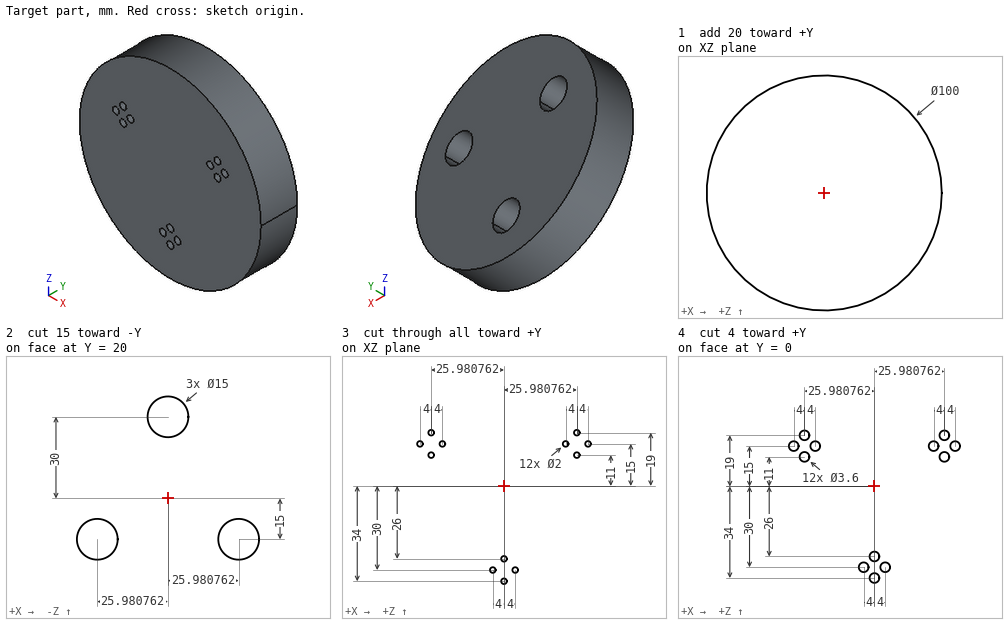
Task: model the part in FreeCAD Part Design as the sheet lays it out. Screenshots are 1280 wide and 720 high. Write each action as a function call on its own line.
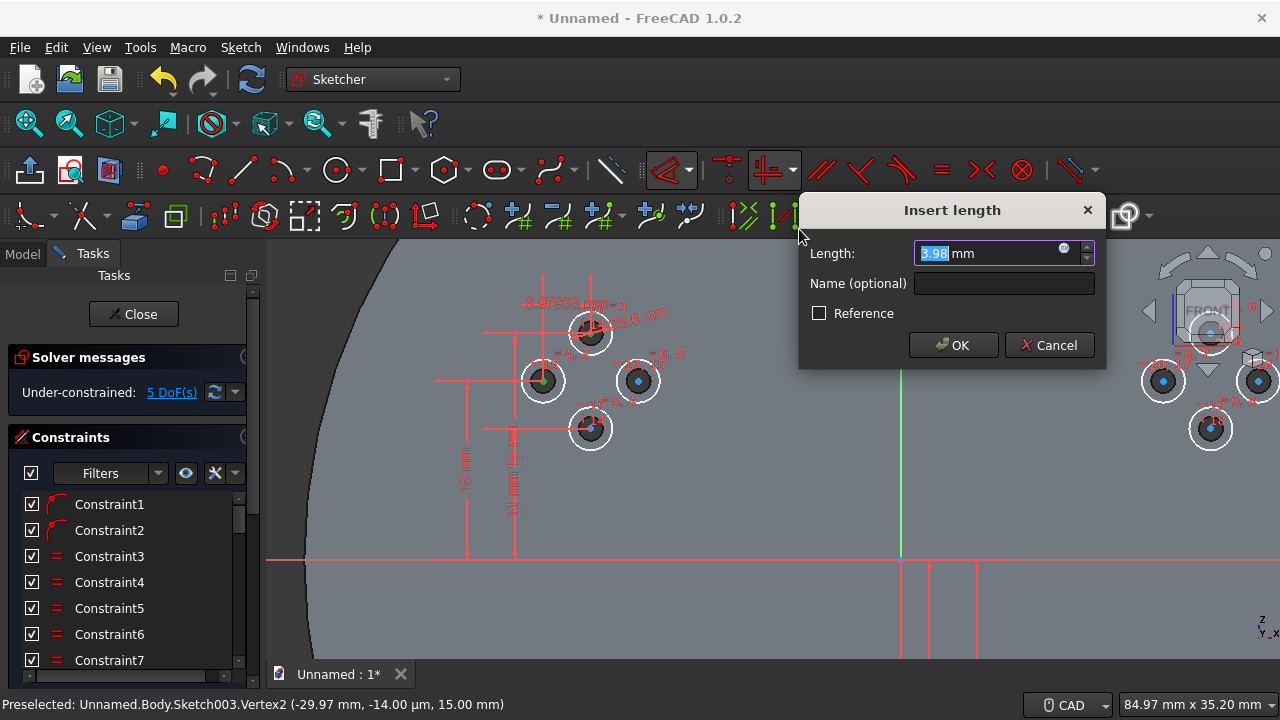
text(4)
key(Return)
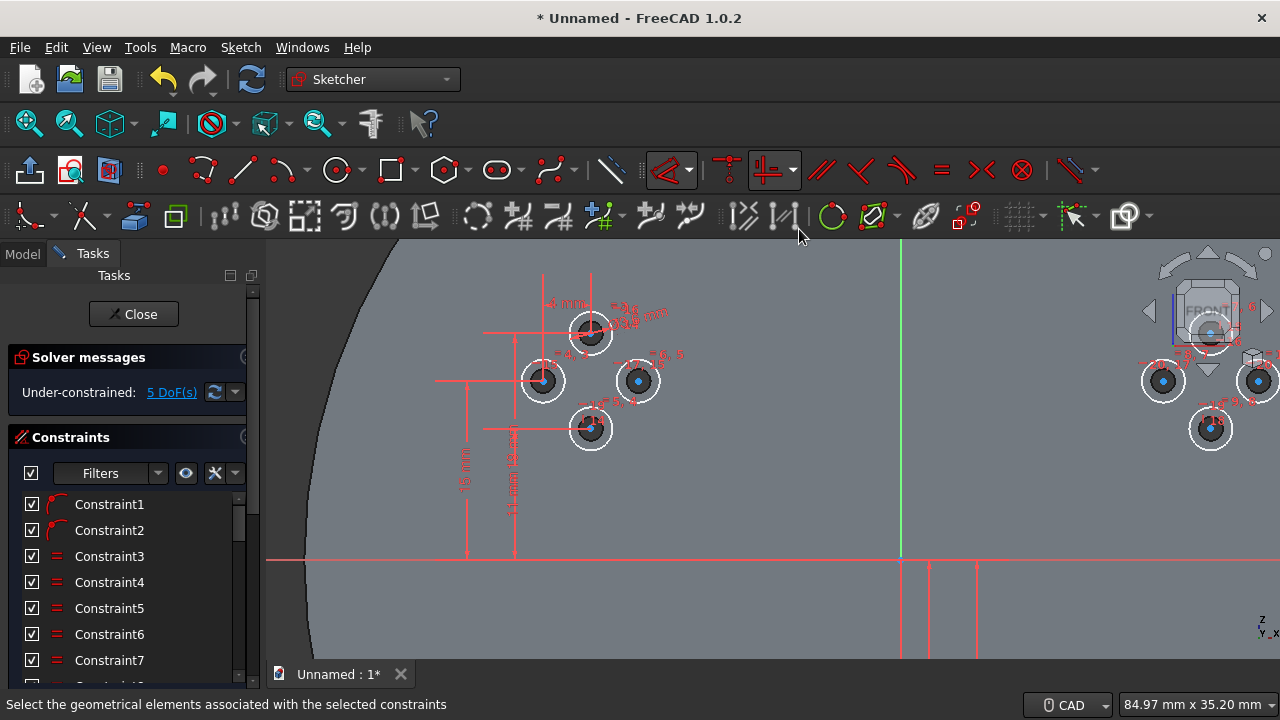
click(591, 333)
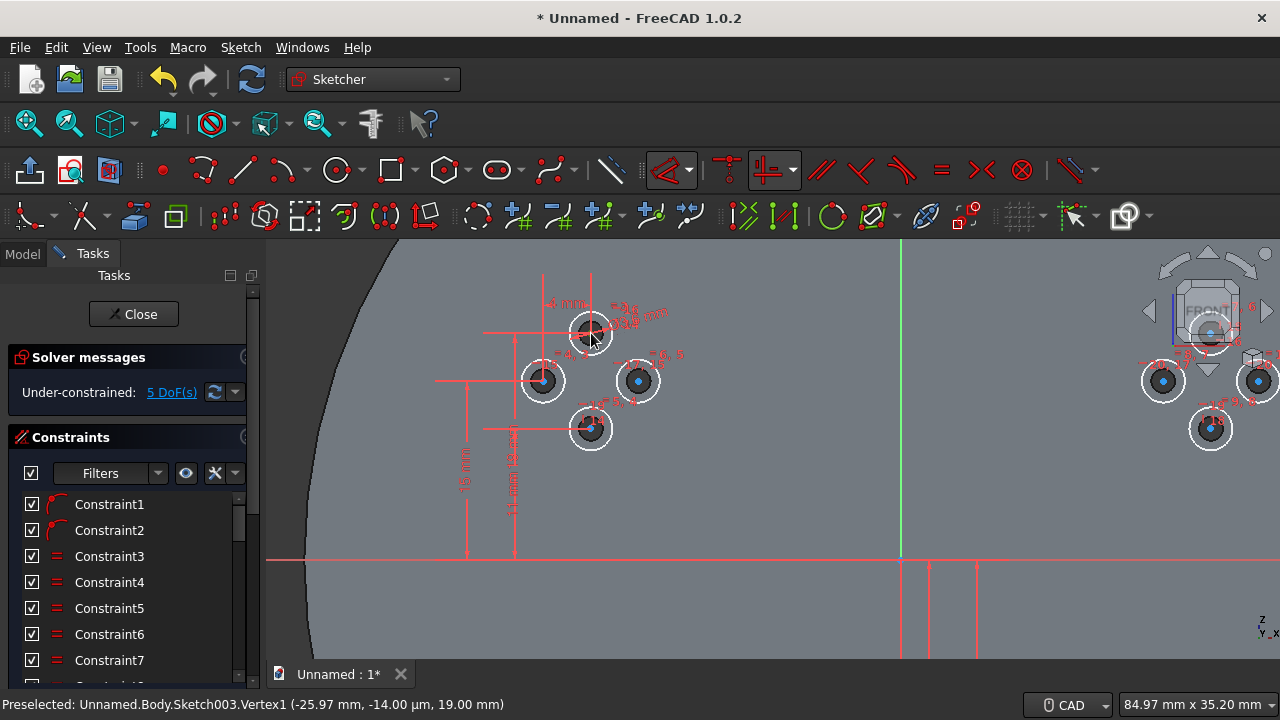
click(638, 381)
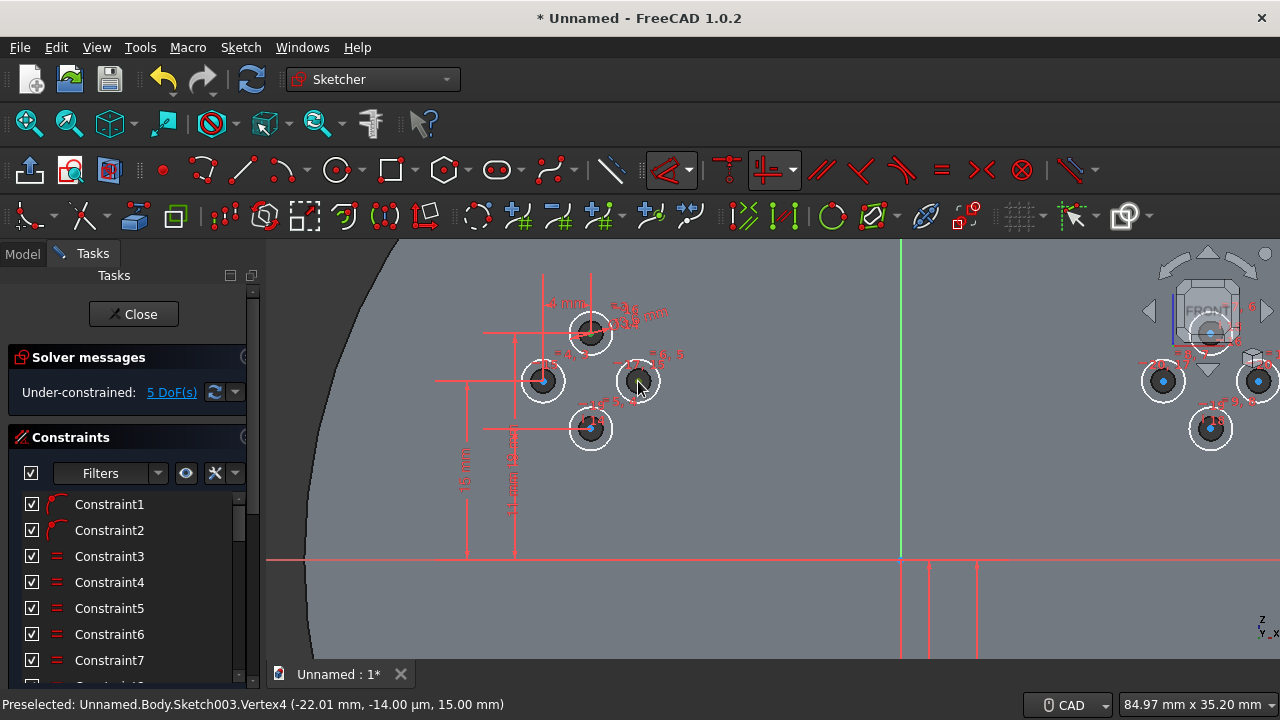
key(l)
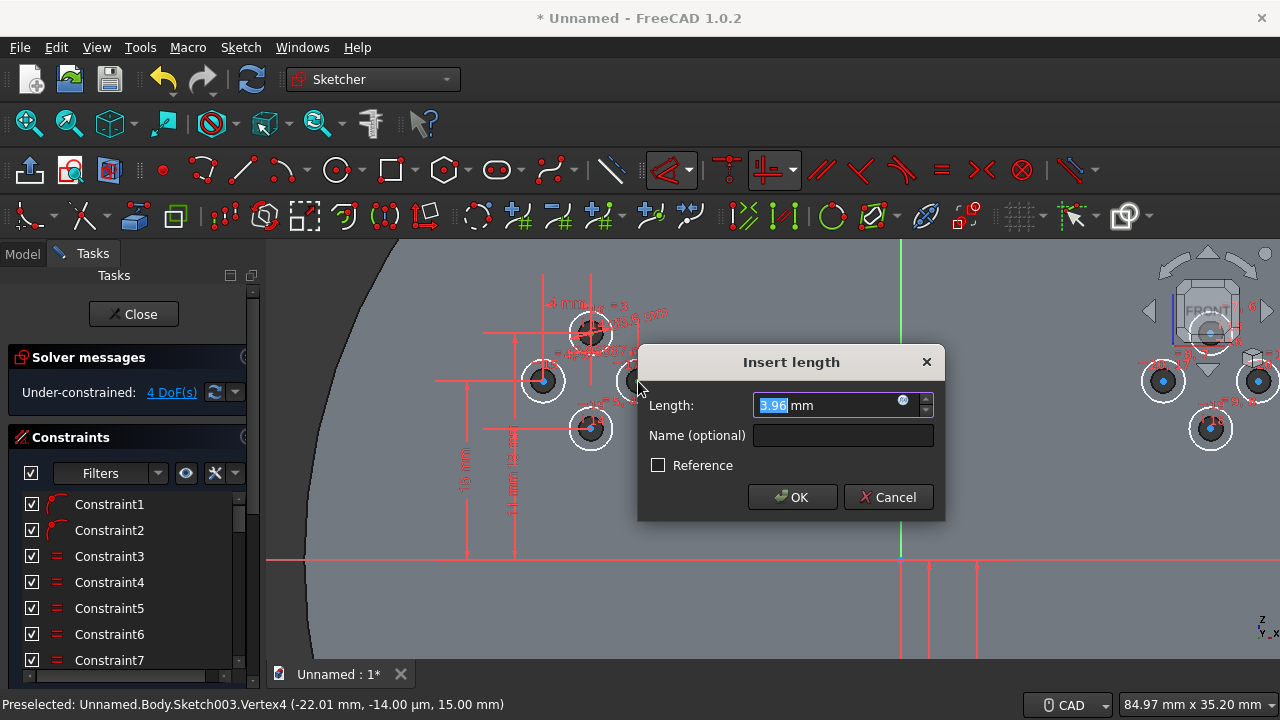
text(4)
key(Return)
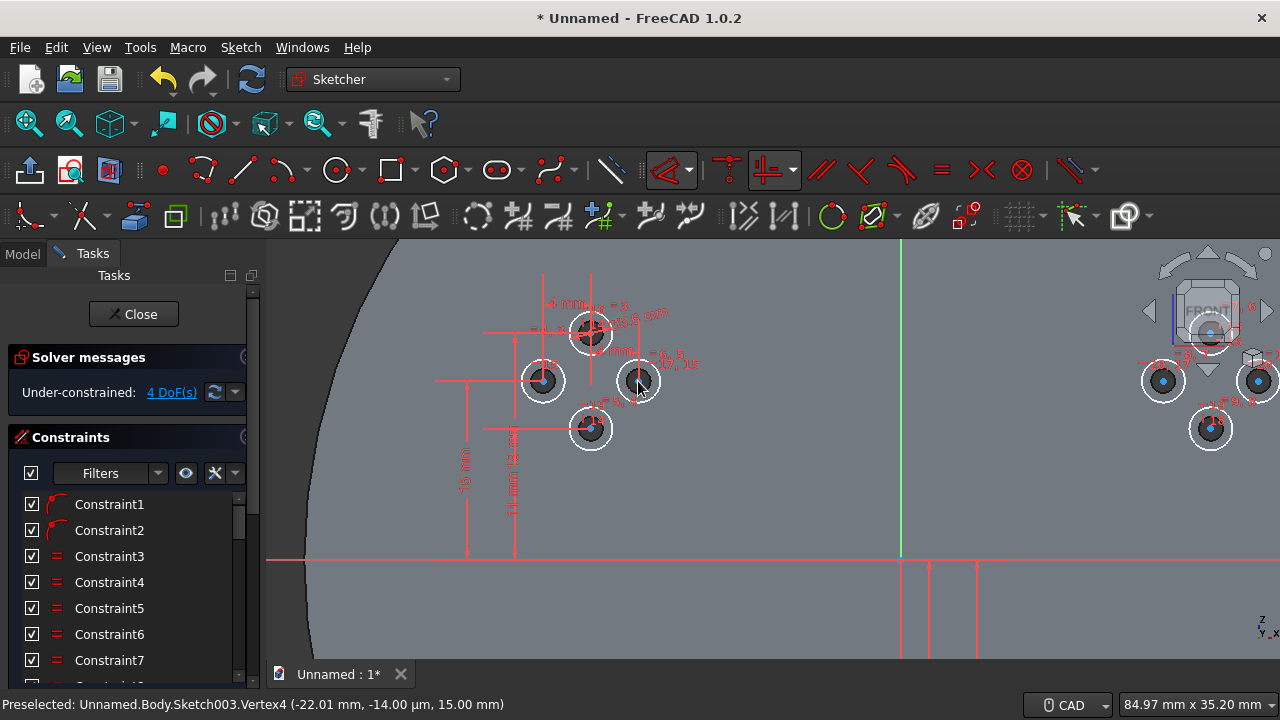
scroll(590, 332, down, 5)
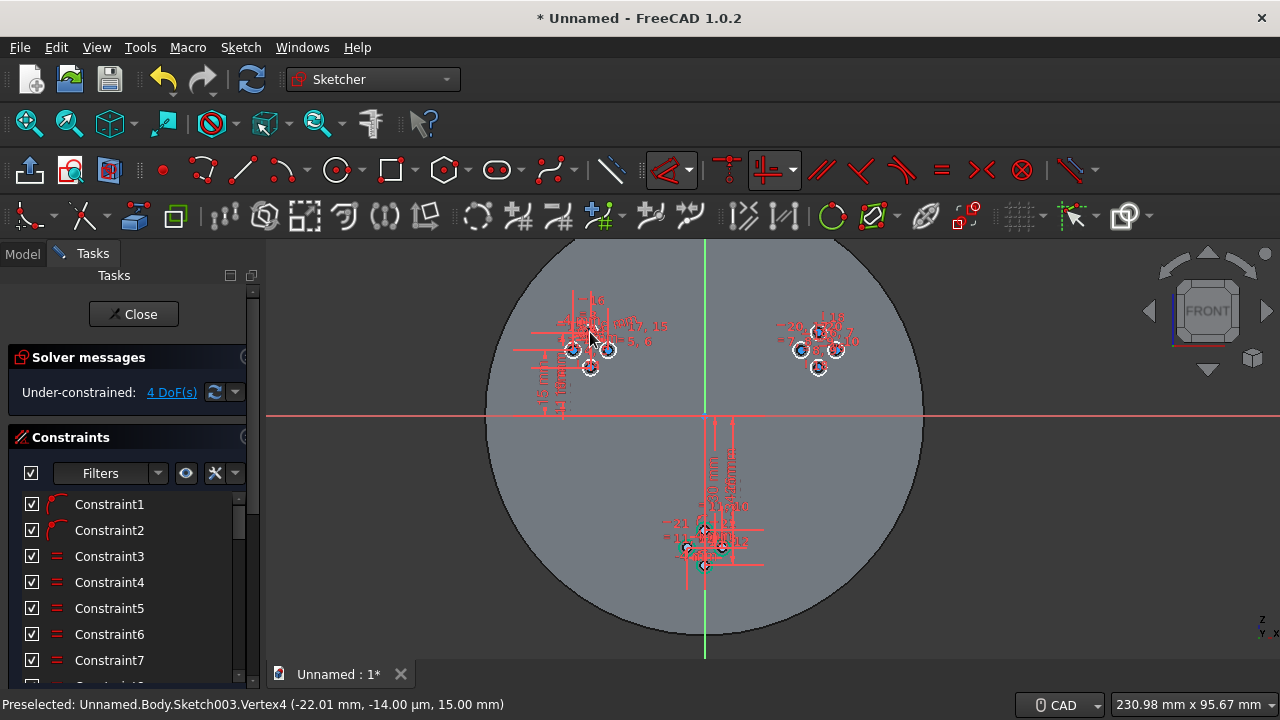
scroll(819, 333, up, 5)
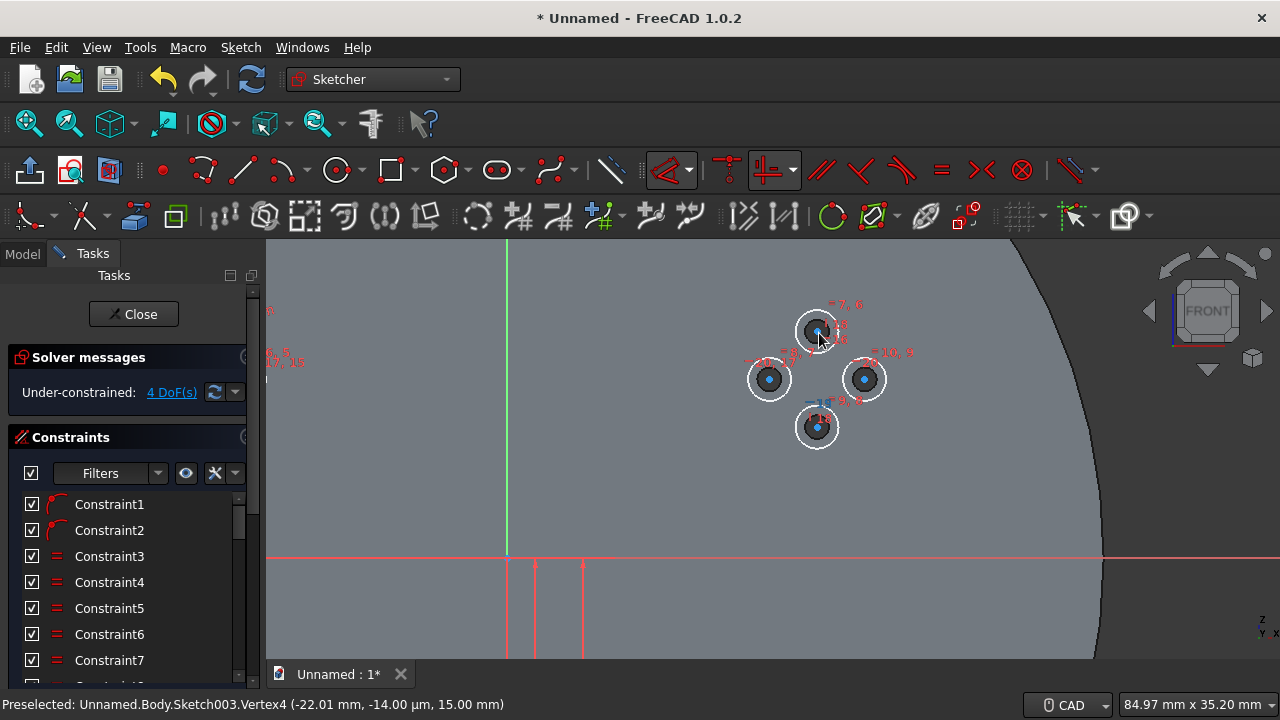
click(817, 332)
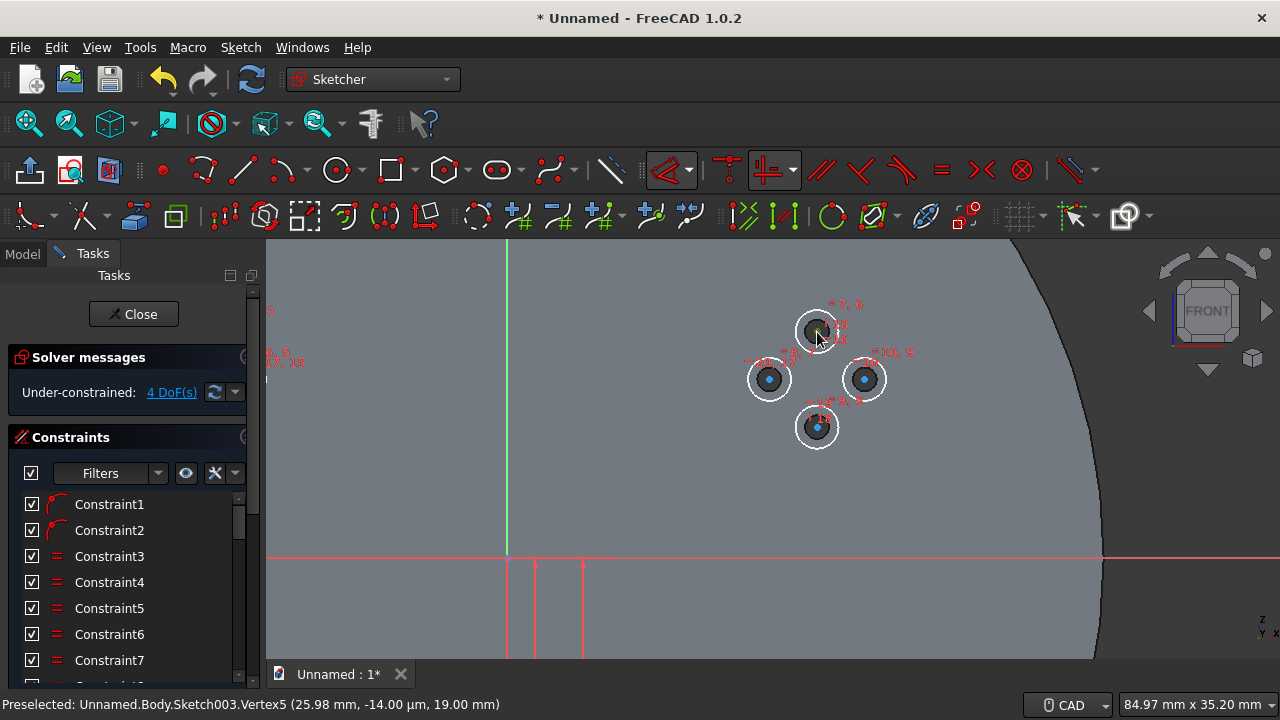
click(770, 379)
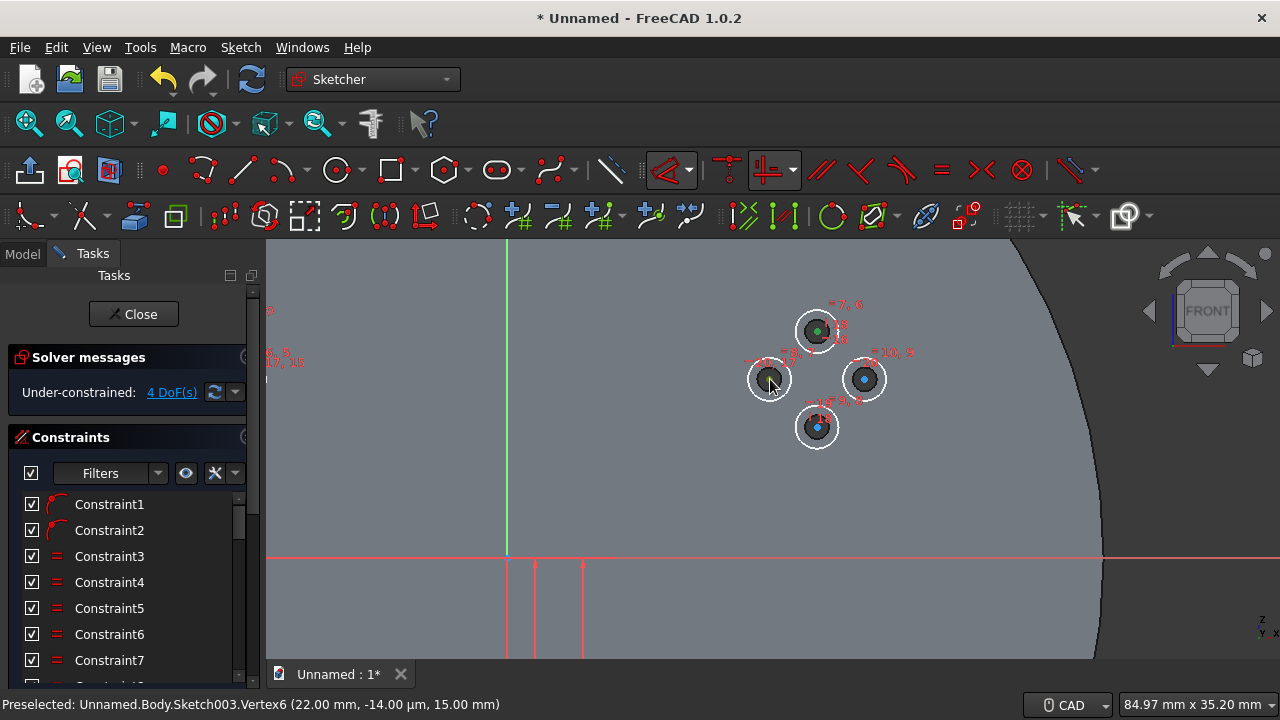
key(l)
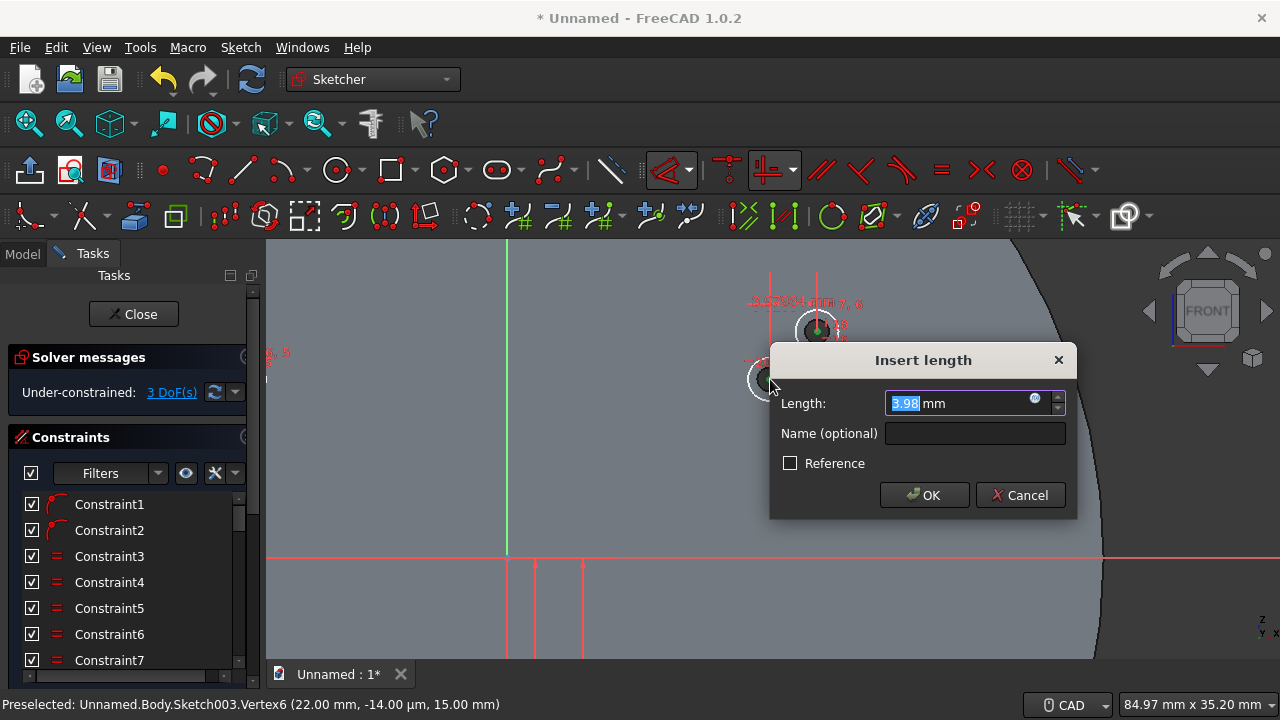
text(4)
key(Return)